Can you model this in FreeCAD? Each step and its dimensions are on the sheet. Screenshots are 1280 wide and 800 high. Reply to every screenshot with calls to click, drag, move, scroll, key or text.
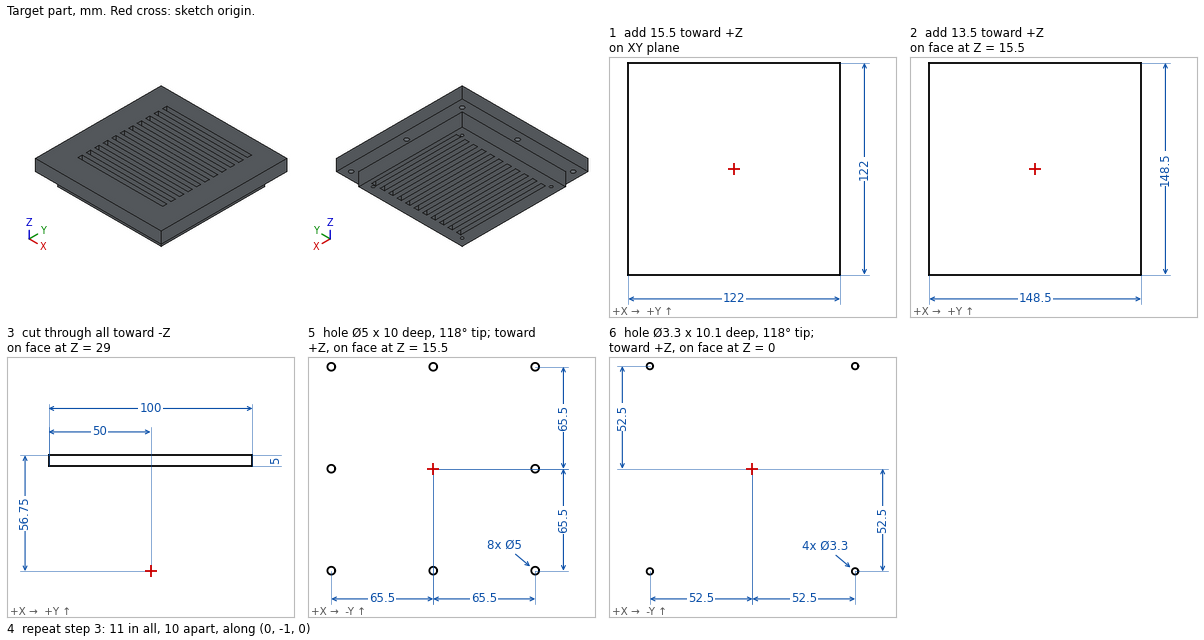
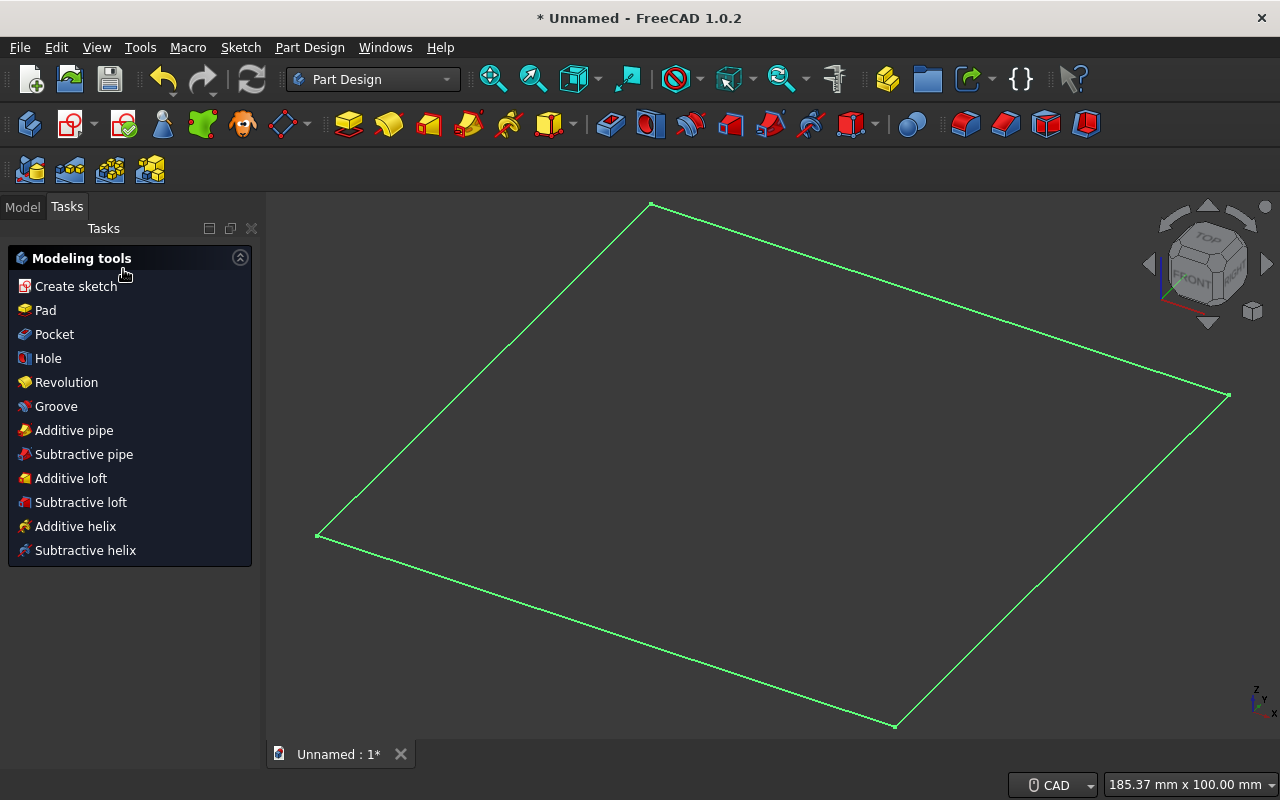
click(350, 124)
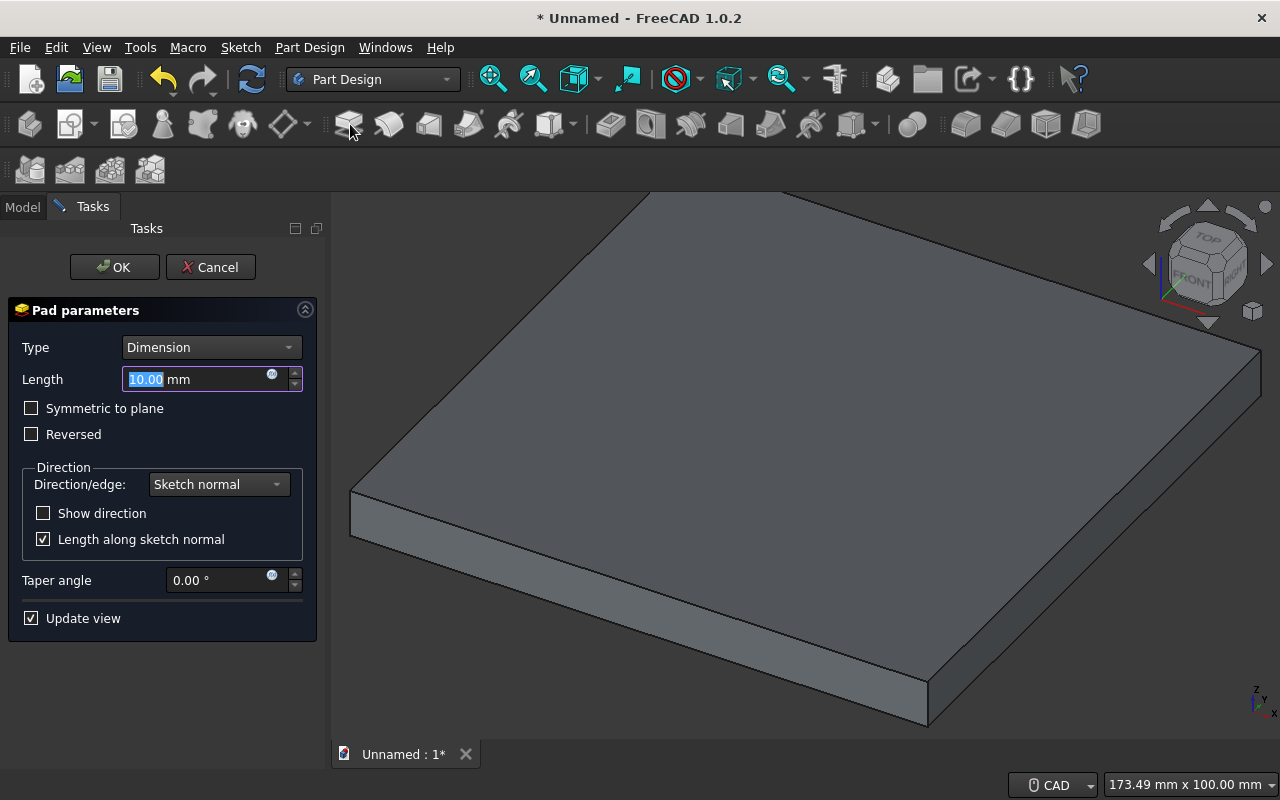
text(15.5)
key(Tab)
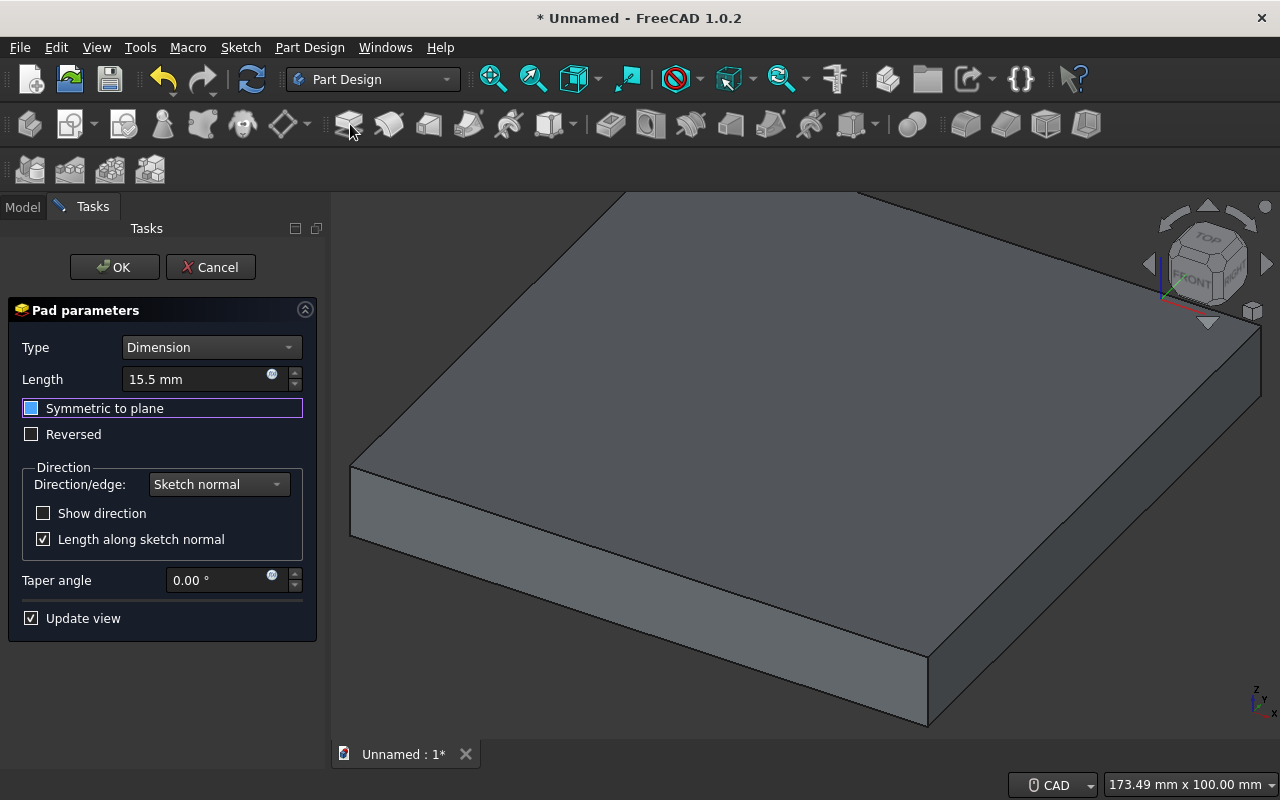
click(115, 267)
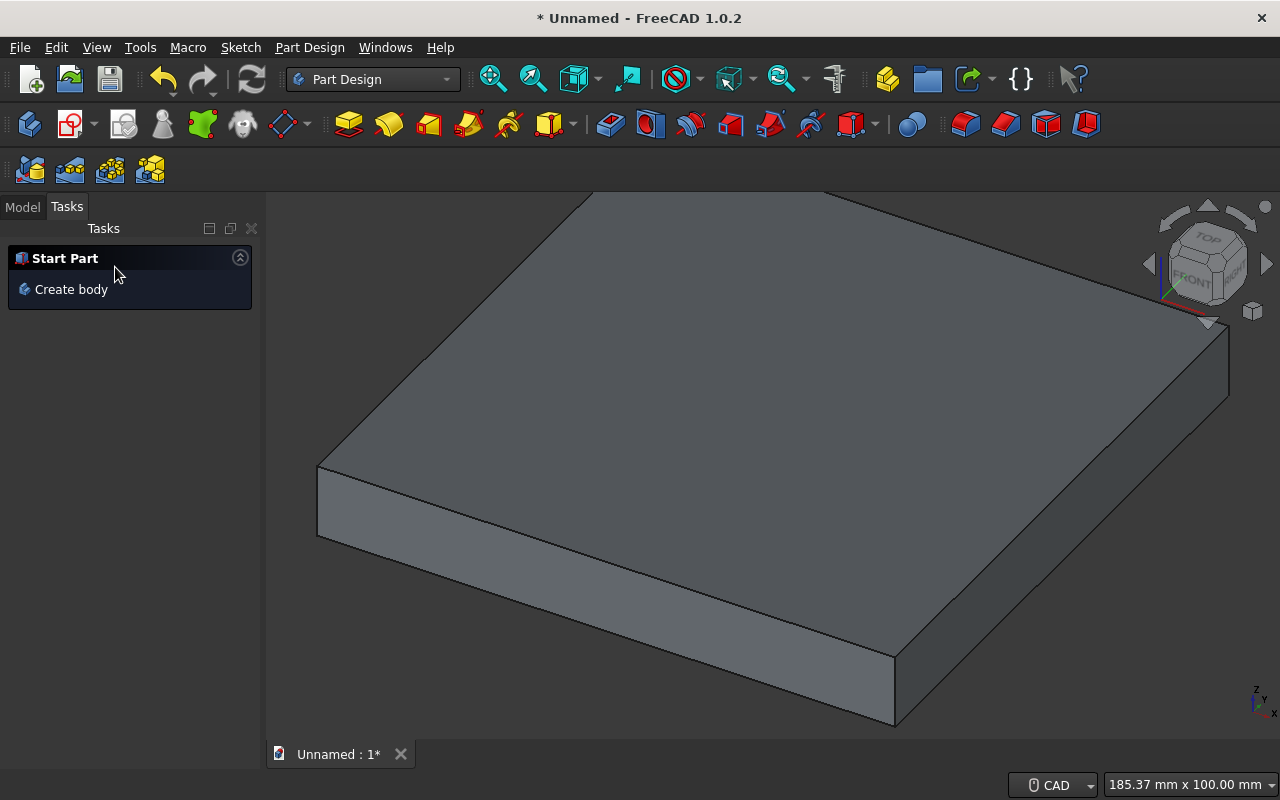
click(494, 80)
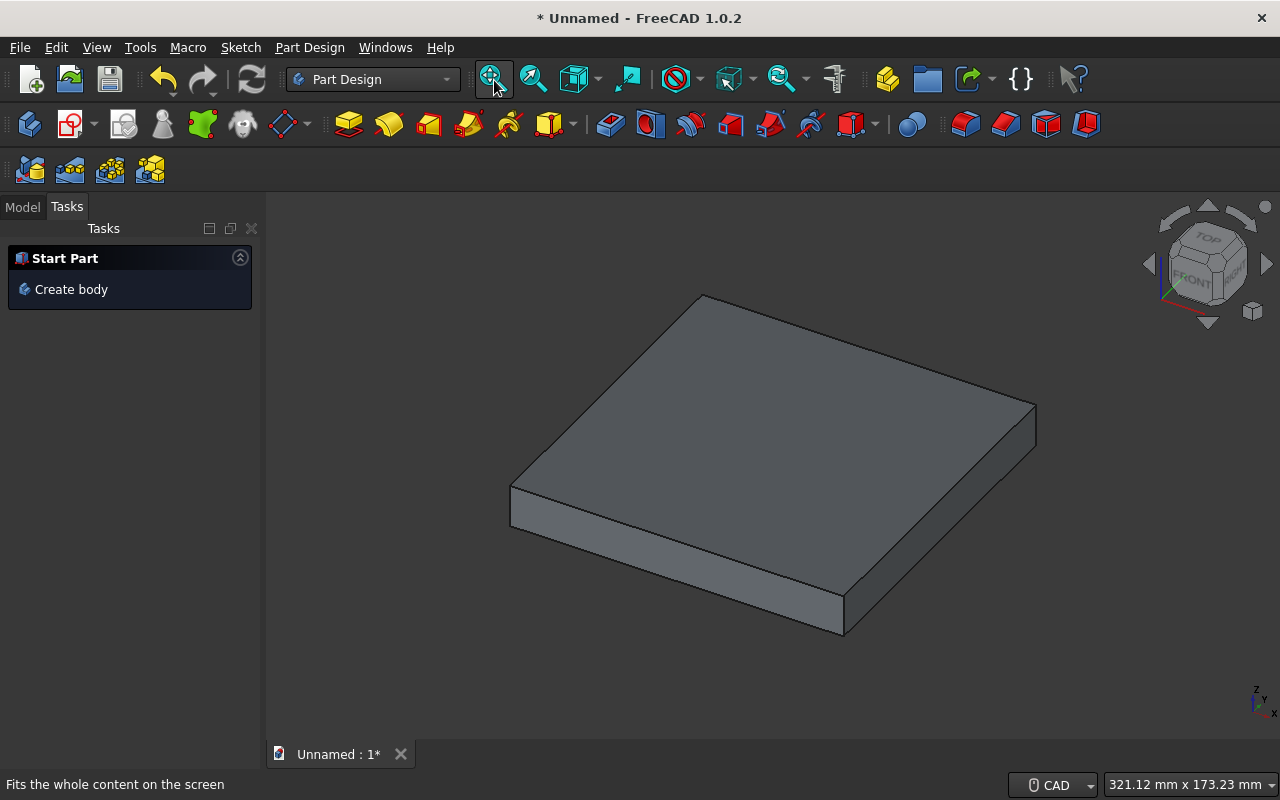
click(773, 444)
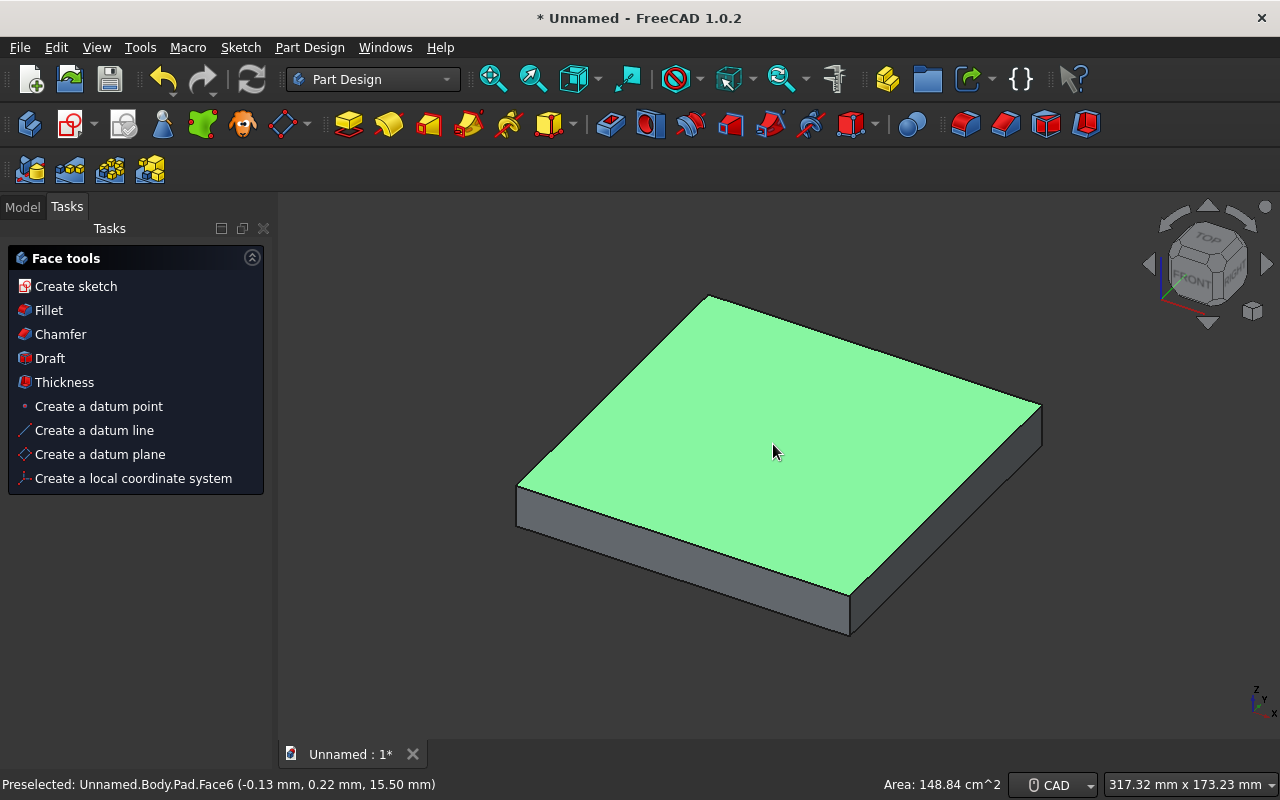
click(70, 124)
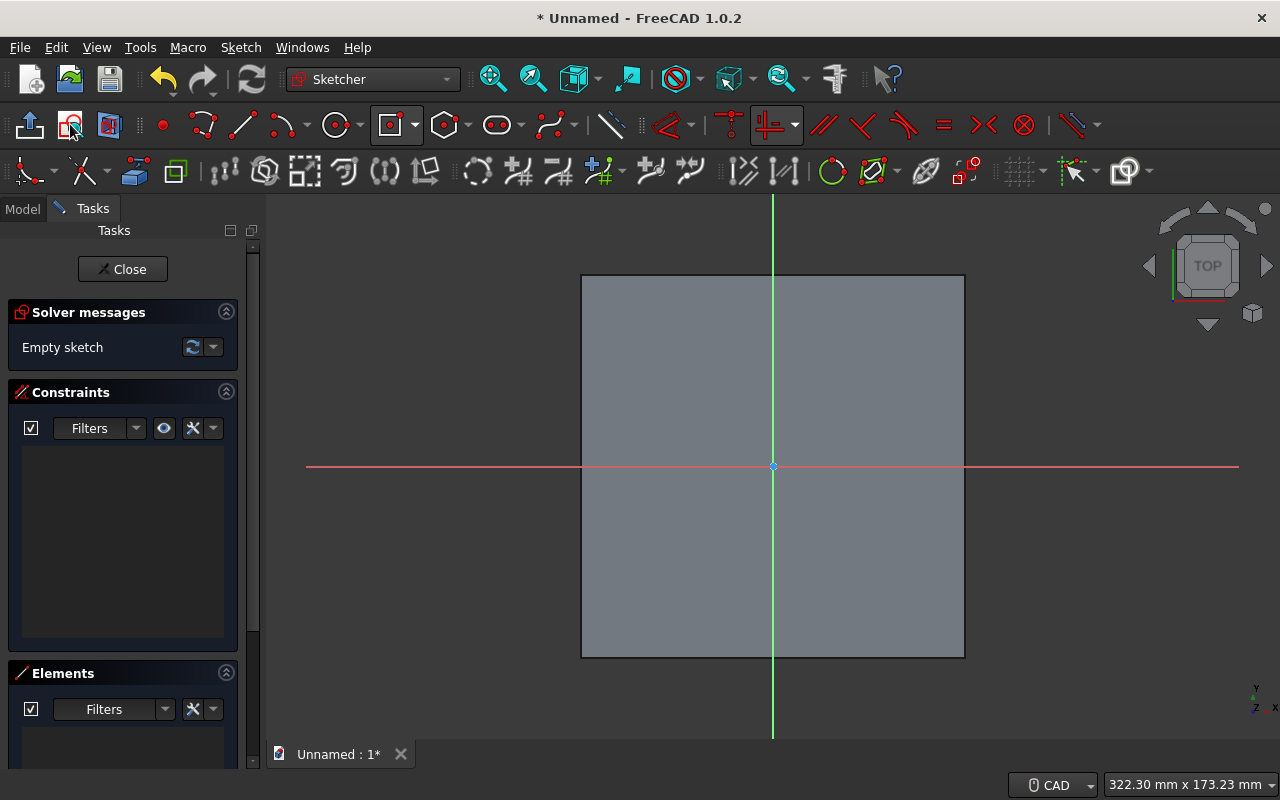
scroll(565, 466, down, 2)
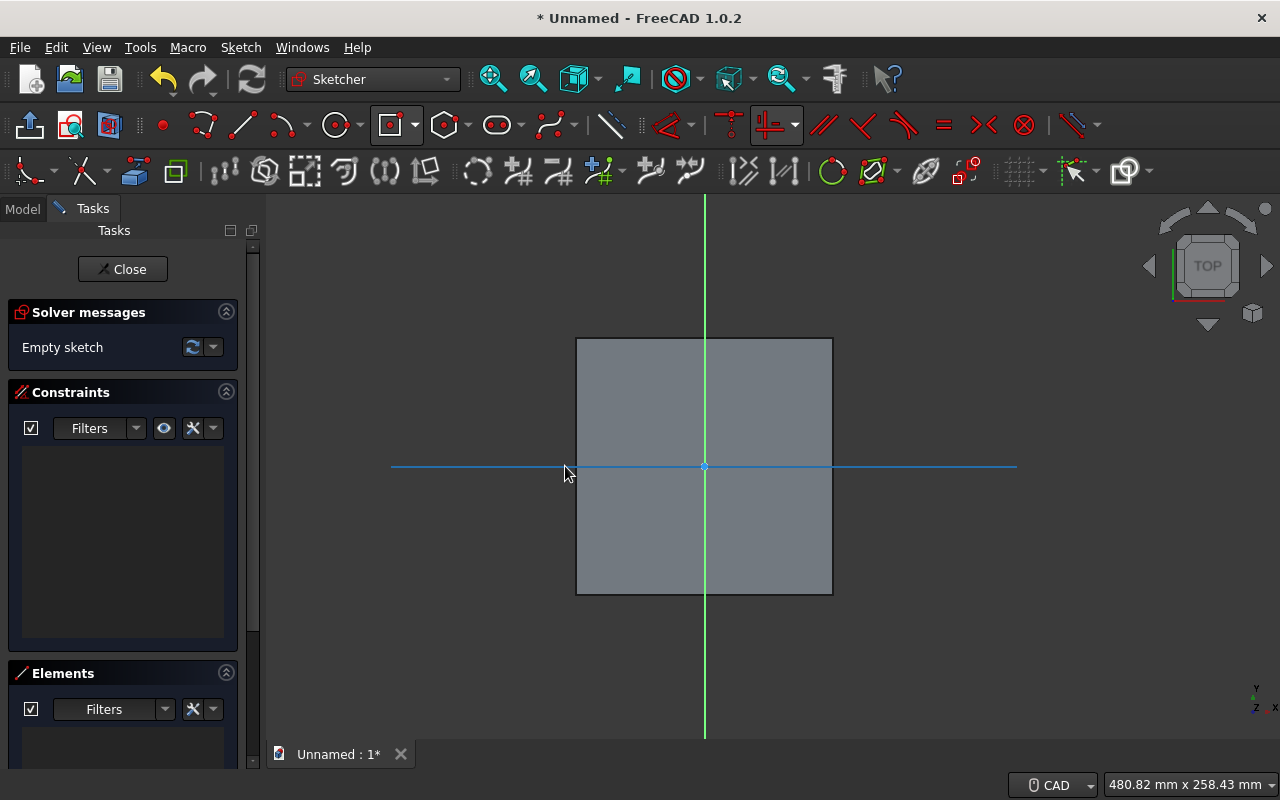
click(390, 126)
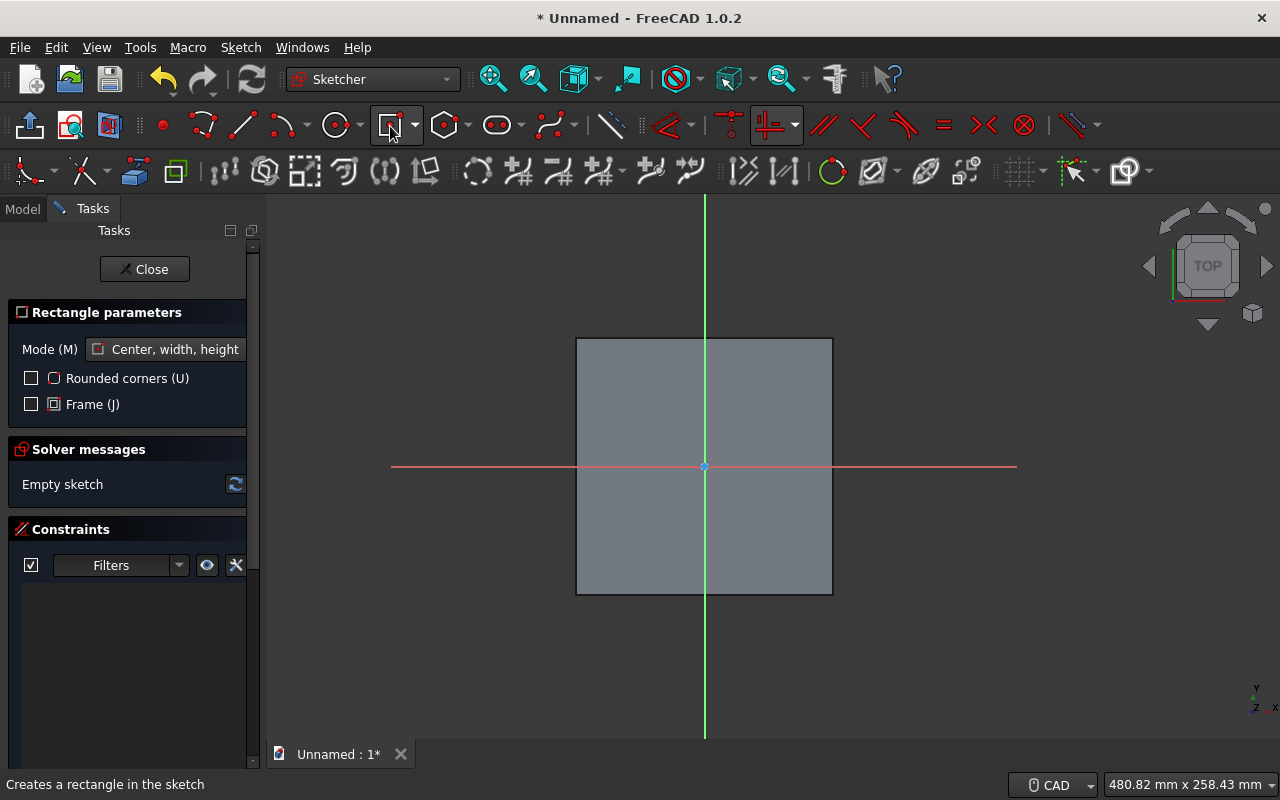
click(705, 466)
move(861, 310)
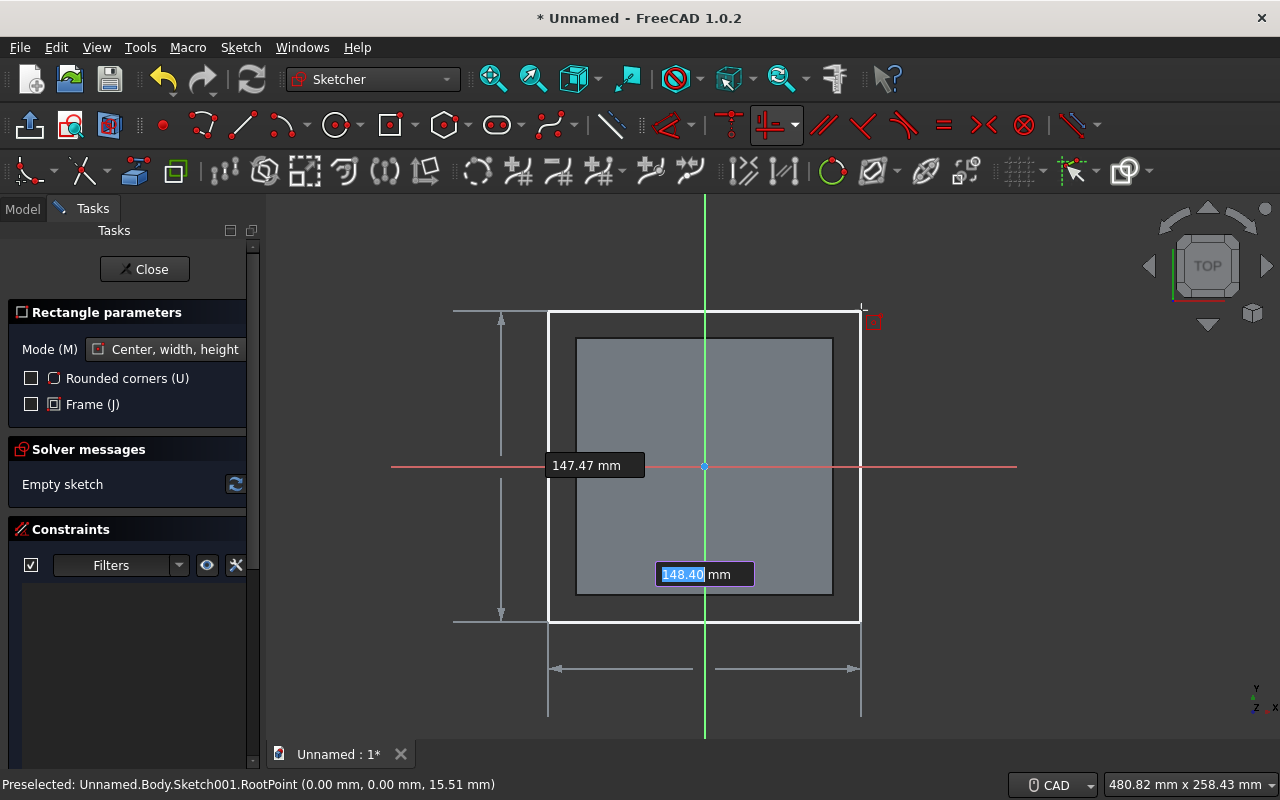
text(148.5)
key(Tab)
text(148.5)
key(Return)
key(Escape)